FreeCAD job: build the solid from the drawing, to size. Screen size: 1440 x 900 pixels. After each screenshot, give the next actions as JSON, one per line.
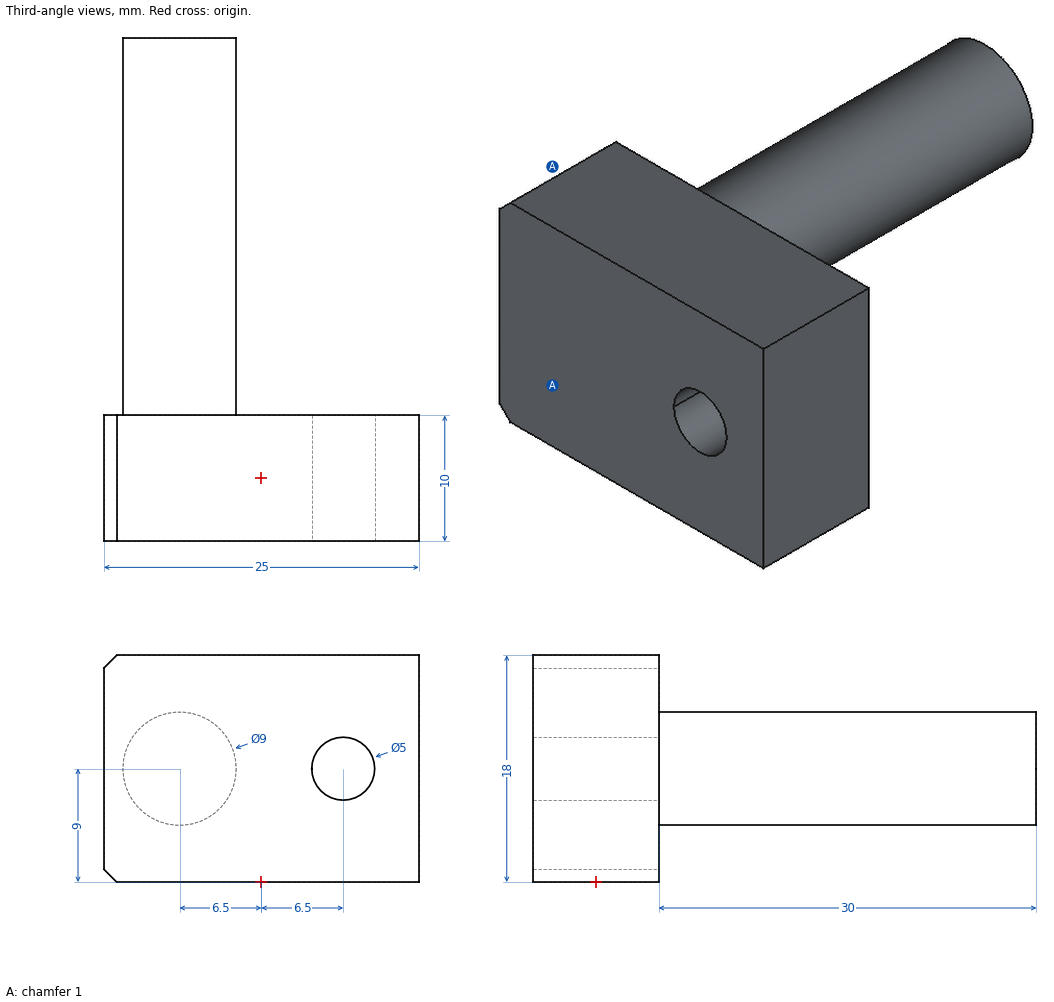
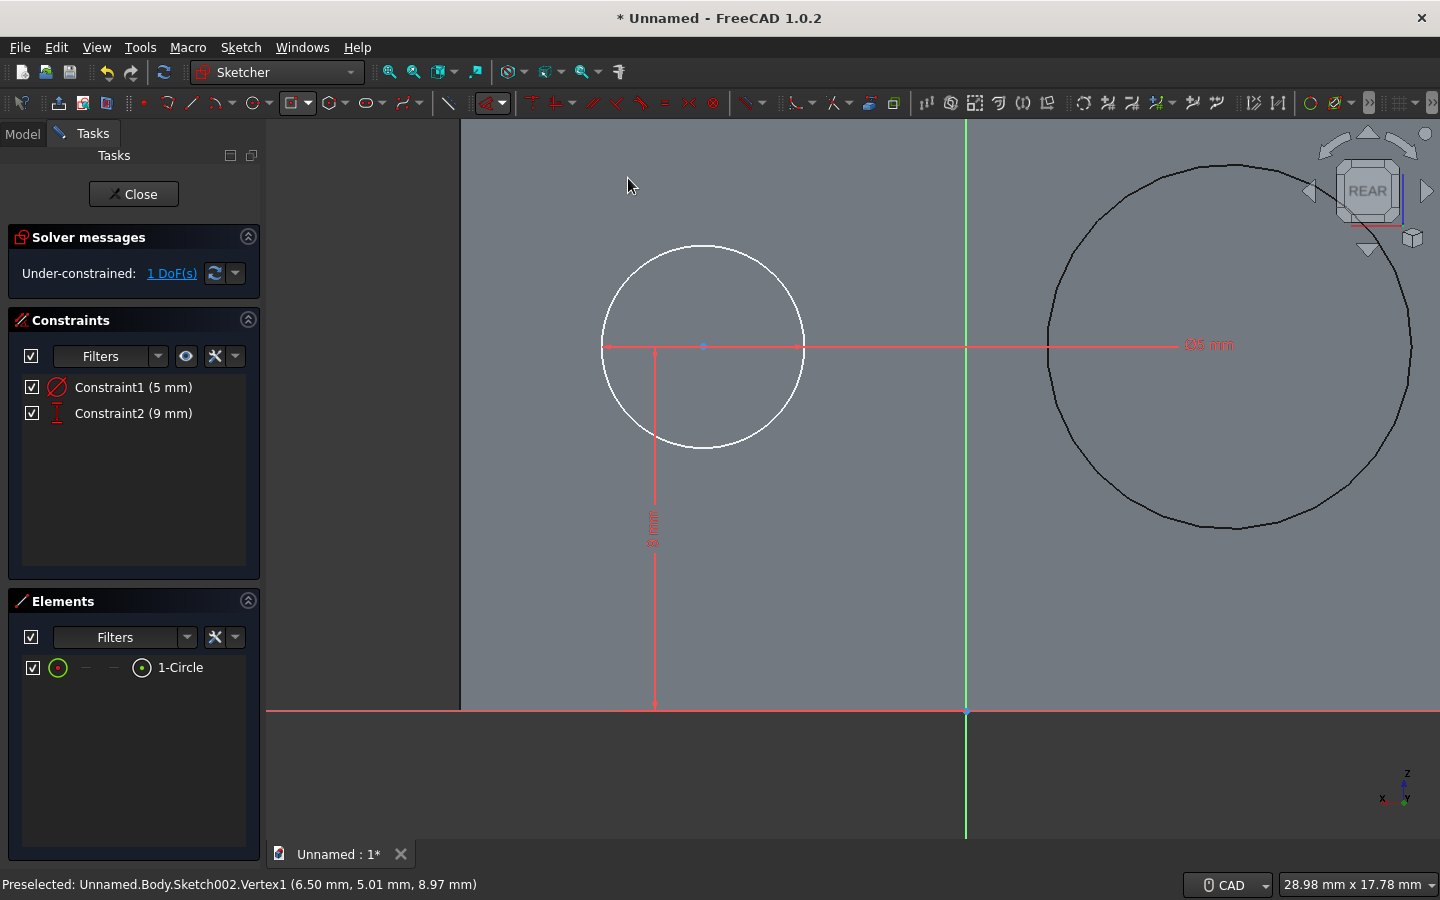
{"action": "left_click", "coordinate": [703, 347]}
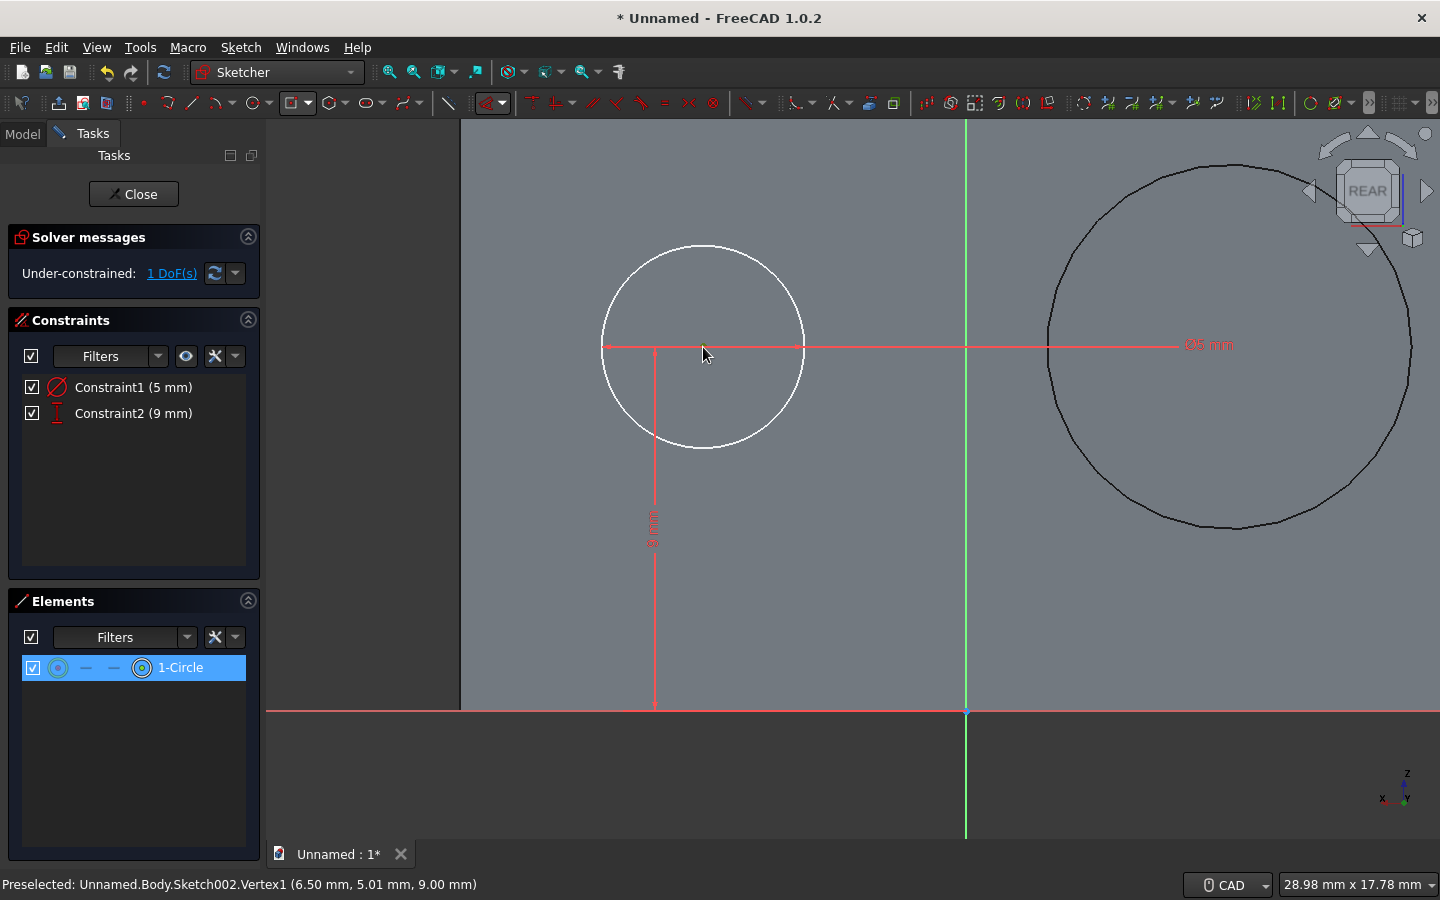
{"action": "key", "text": "l"}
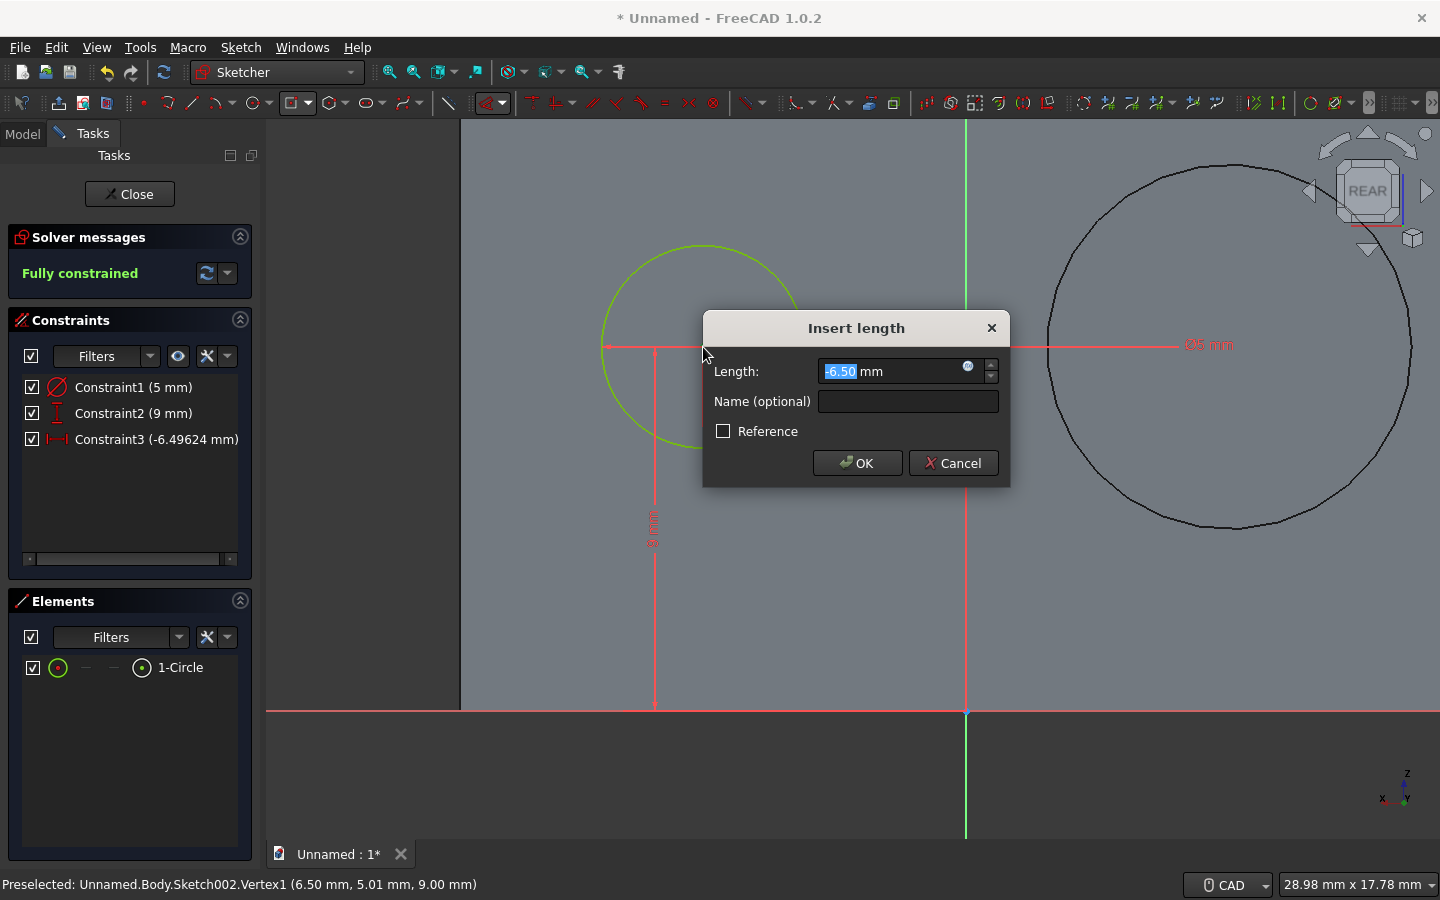
{"action": "type", "text": "-6.5"}
{"action": "key", "text": "Return"}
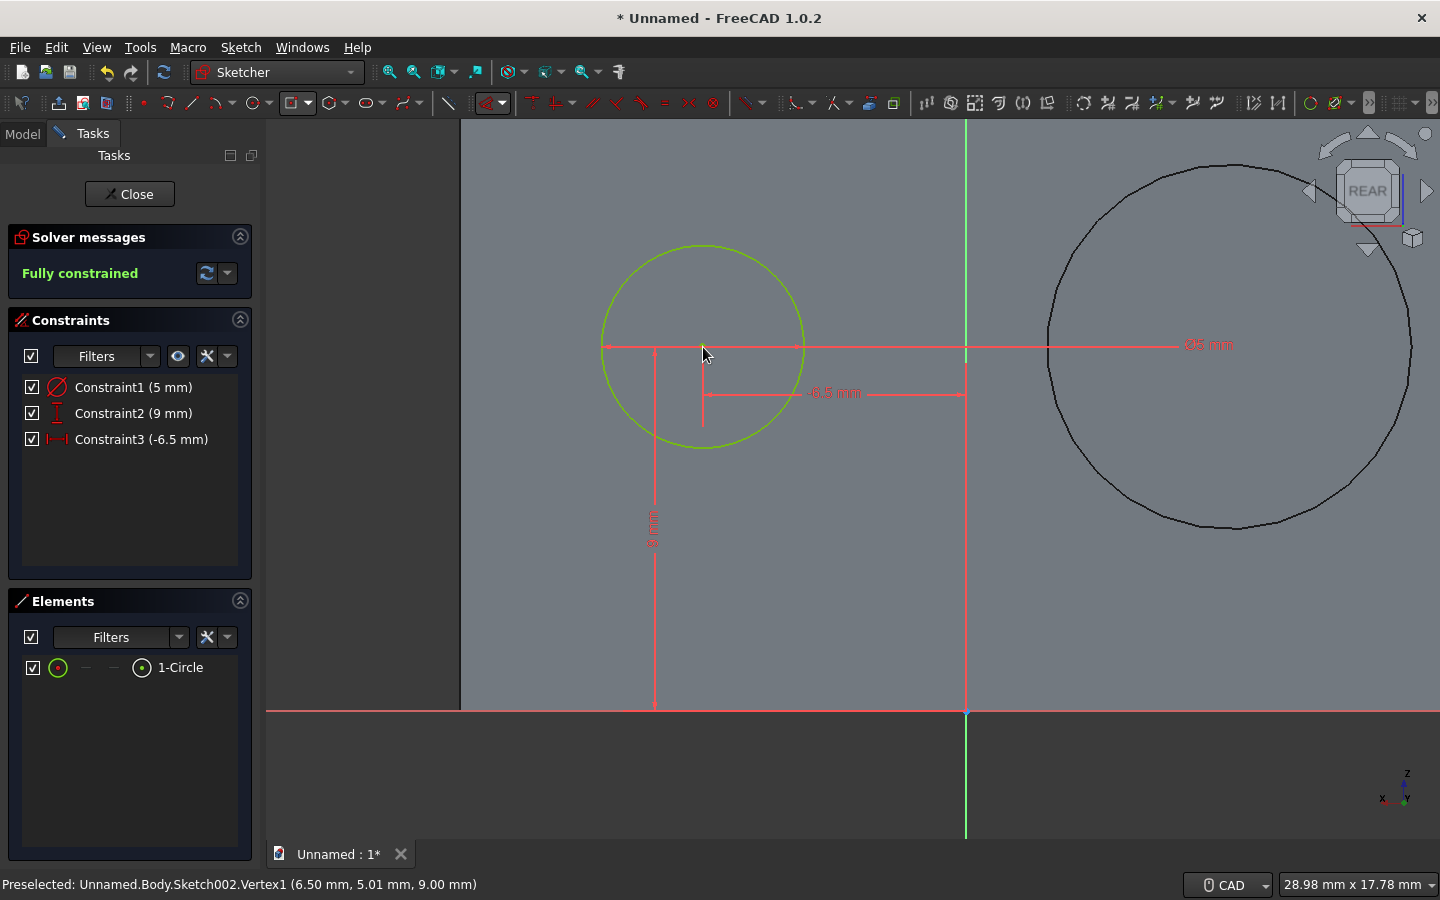
{"action": "left_click", "coordinate": [130, 194]}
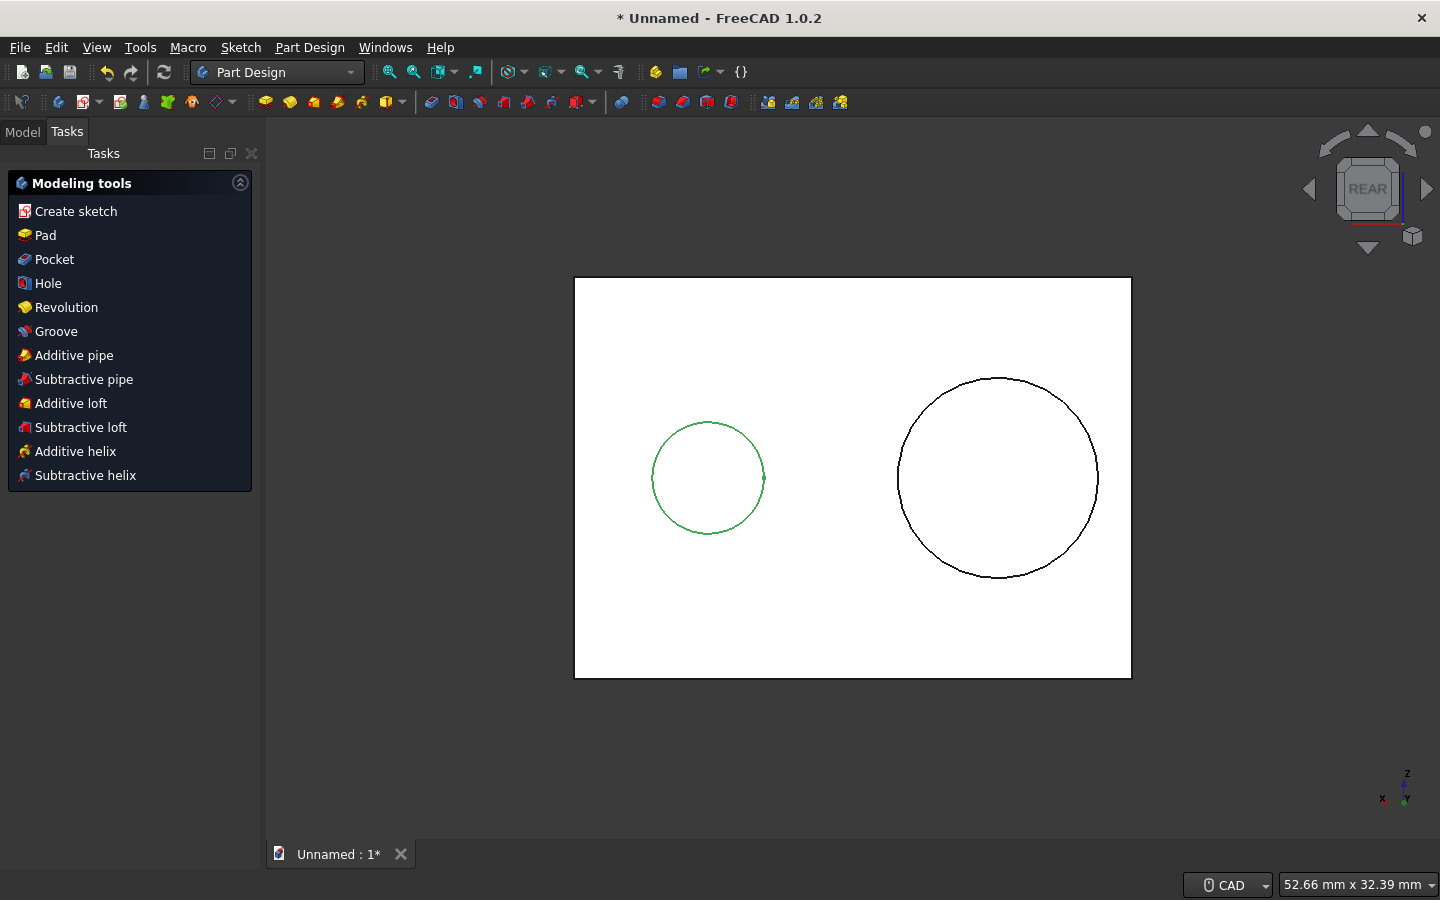
{"action": "left_click", "coordinate": [432, 102]}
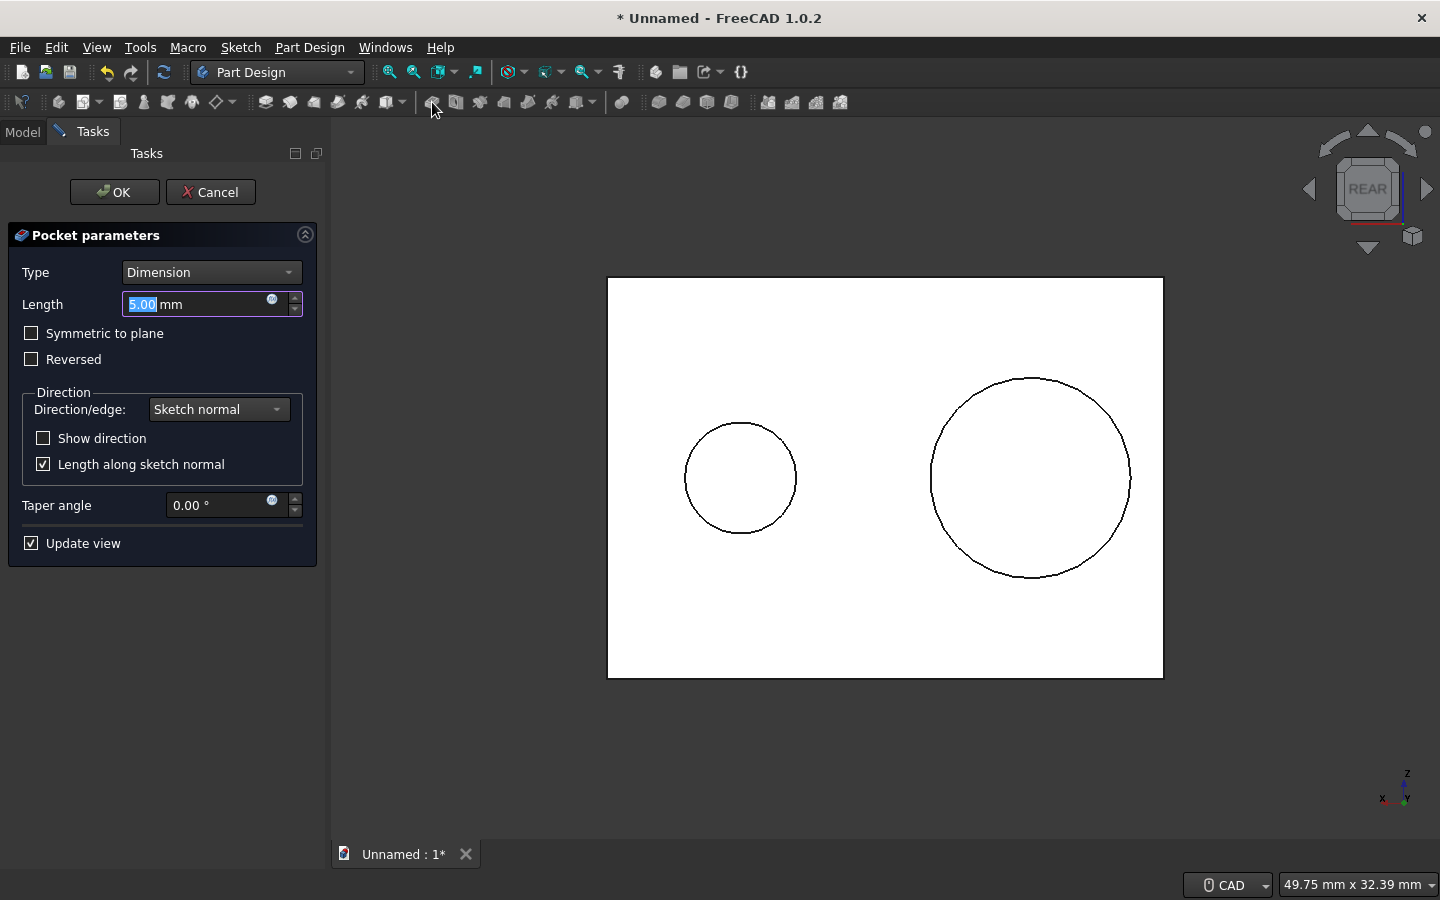
{"action": "left_click", "coordinate": [212, 272]}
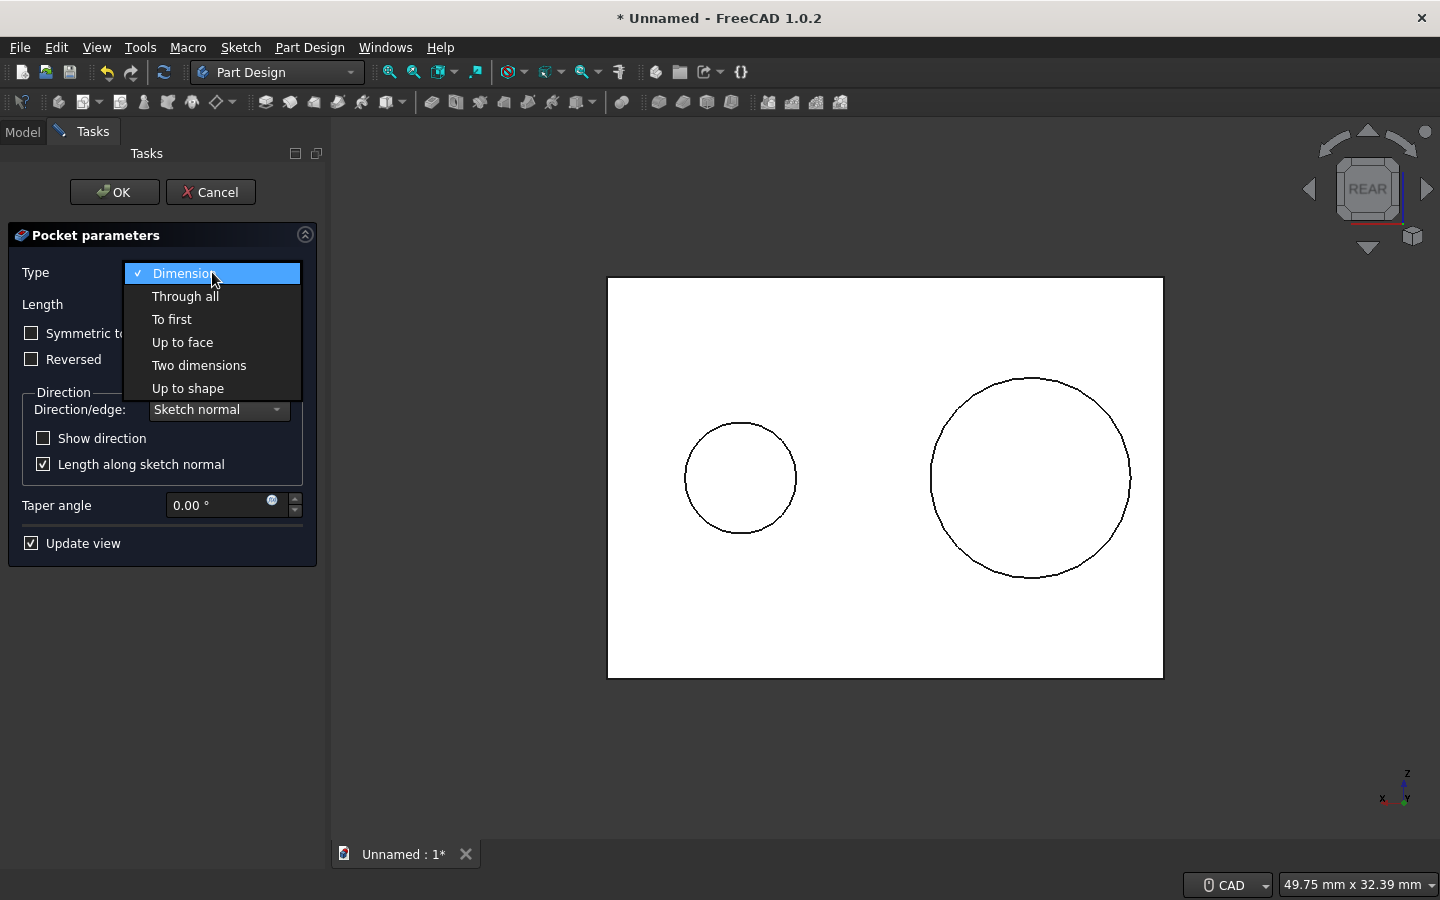
{"action": "left_click", "coordinate": [212, 320]}